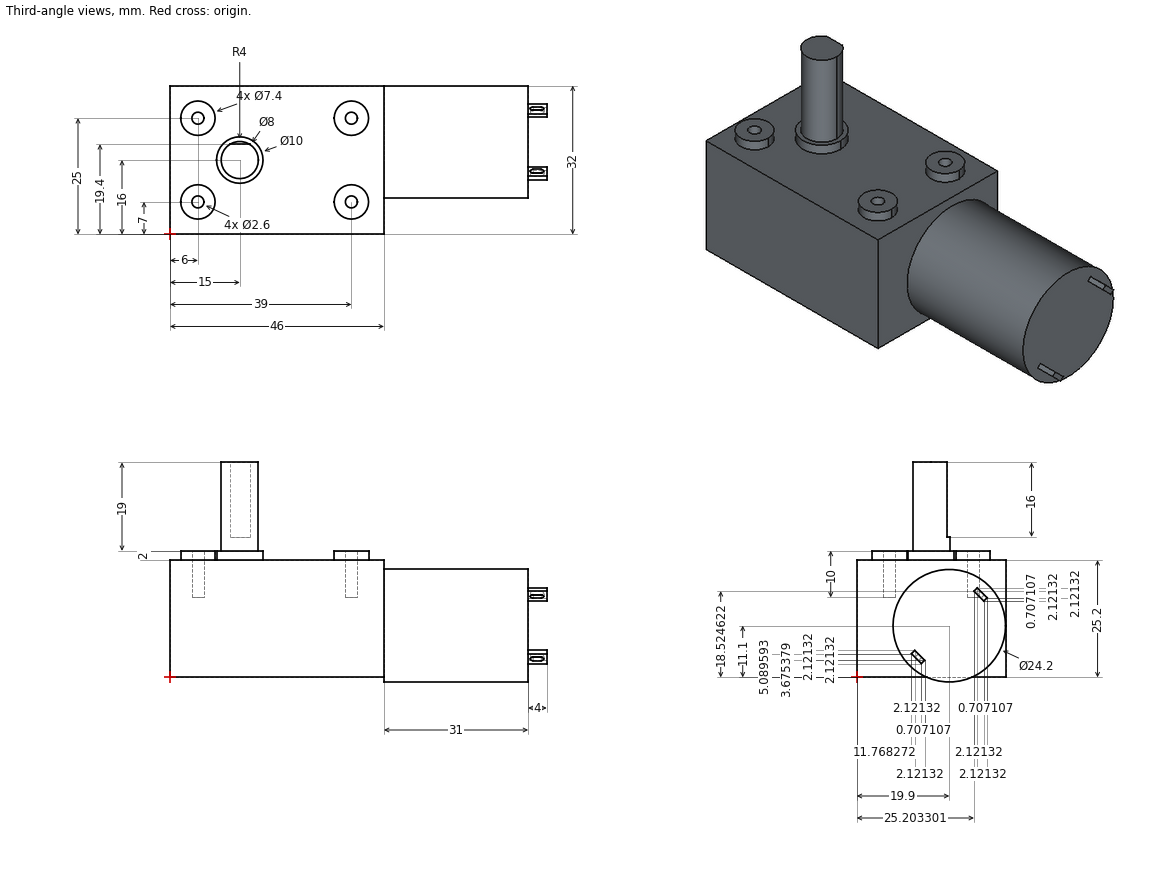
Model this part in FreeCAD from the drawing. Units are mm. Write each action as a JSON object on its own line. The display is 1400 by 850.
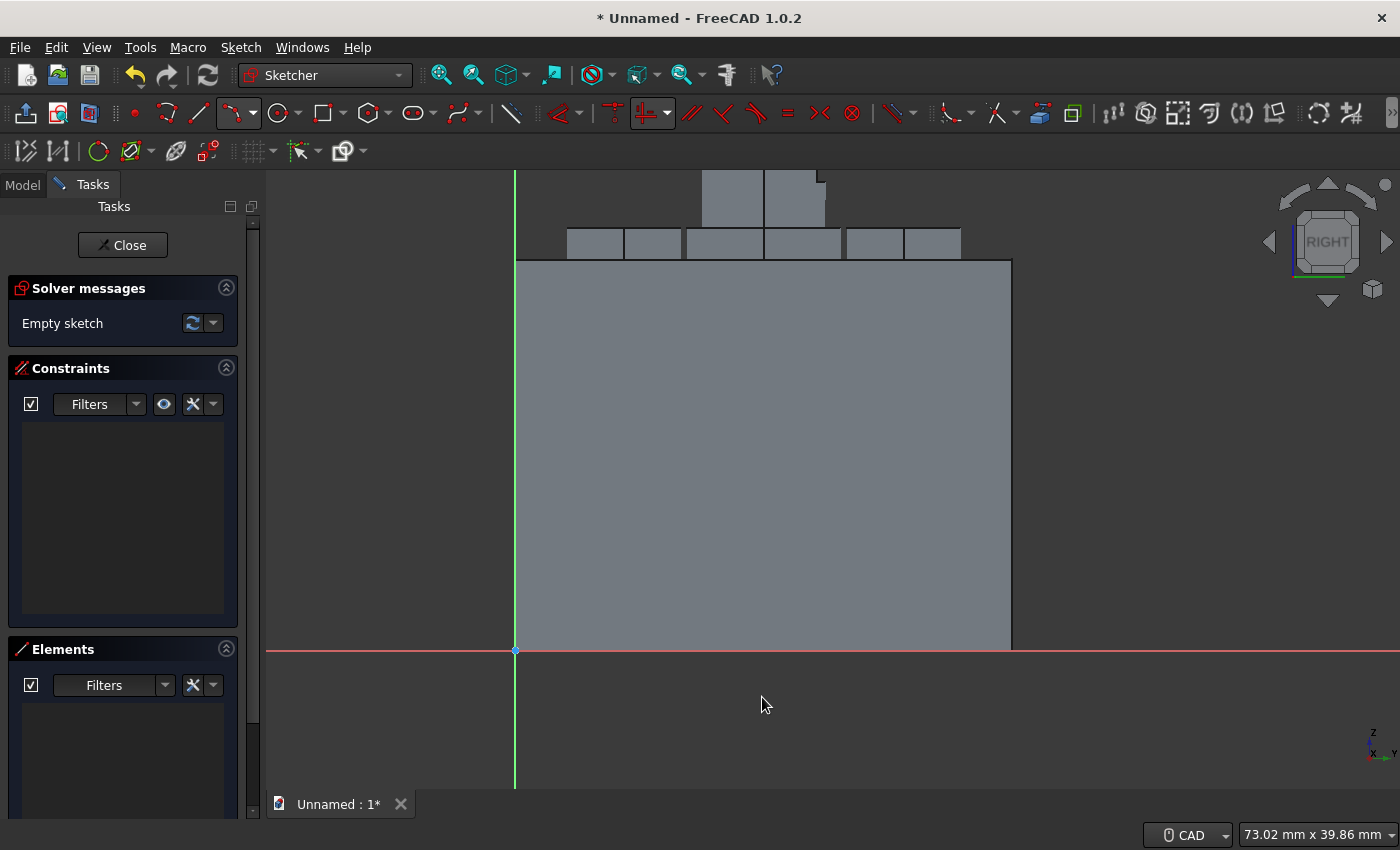
{"action": "left_click", "coordinate": [278, 114]}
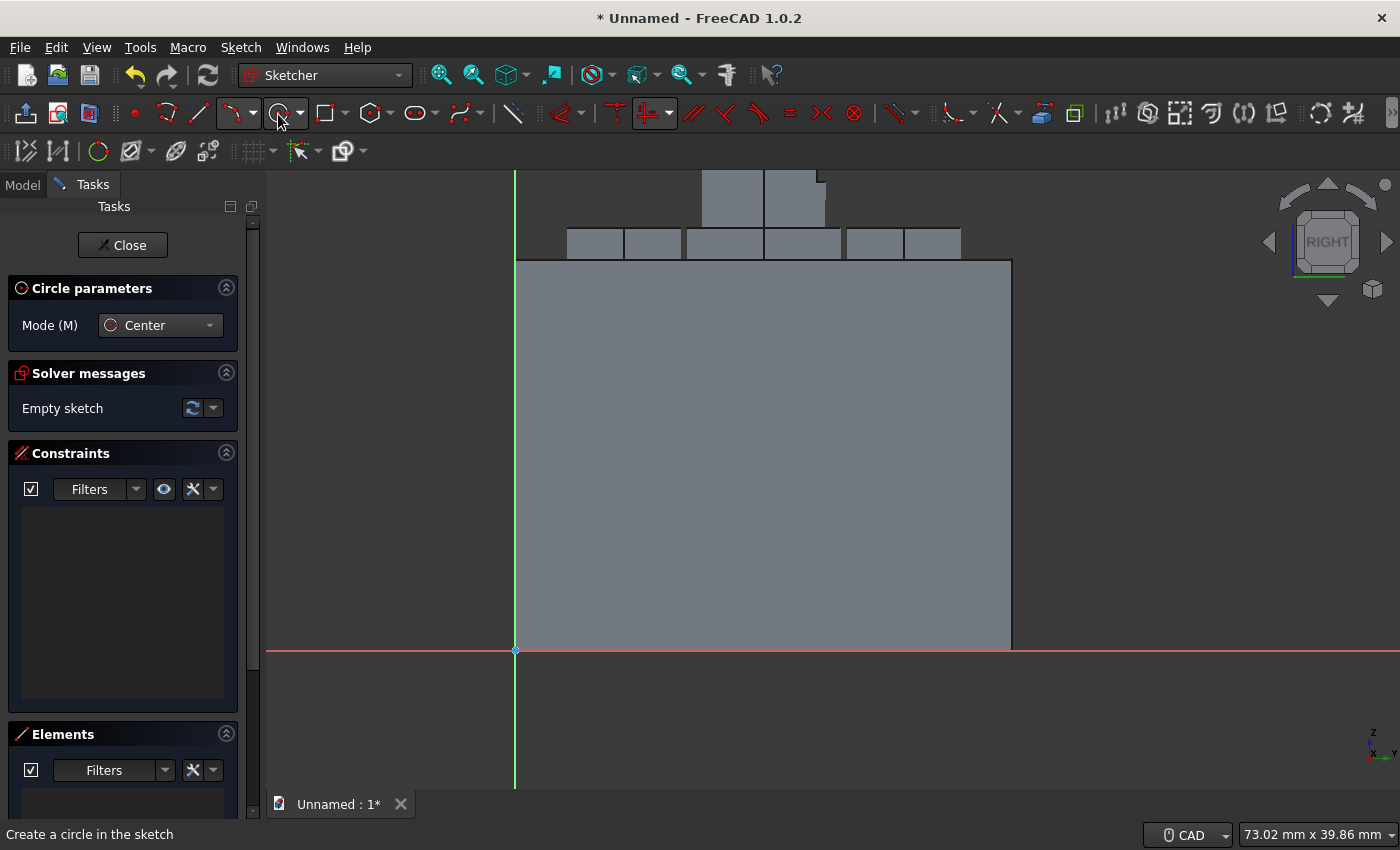
{"action": "left_click", "coordinate": [824, 478]}
{"action": "mouse_move", "coordinate": [957, 346]}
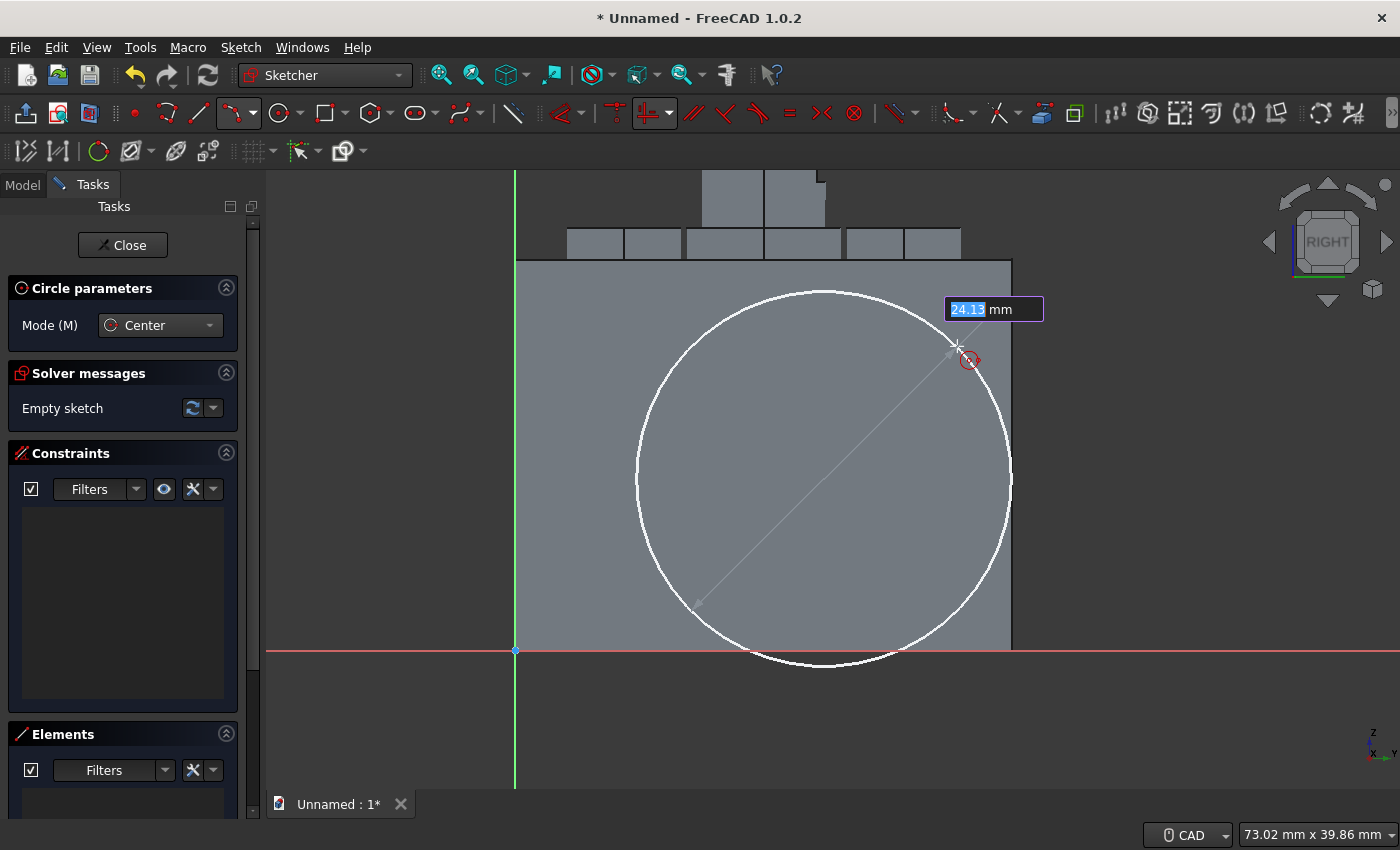
{"action": "type", "text": "24.2"}
{"action": "key", "text": "Return"}
{"action": "key", "text": "Escape"}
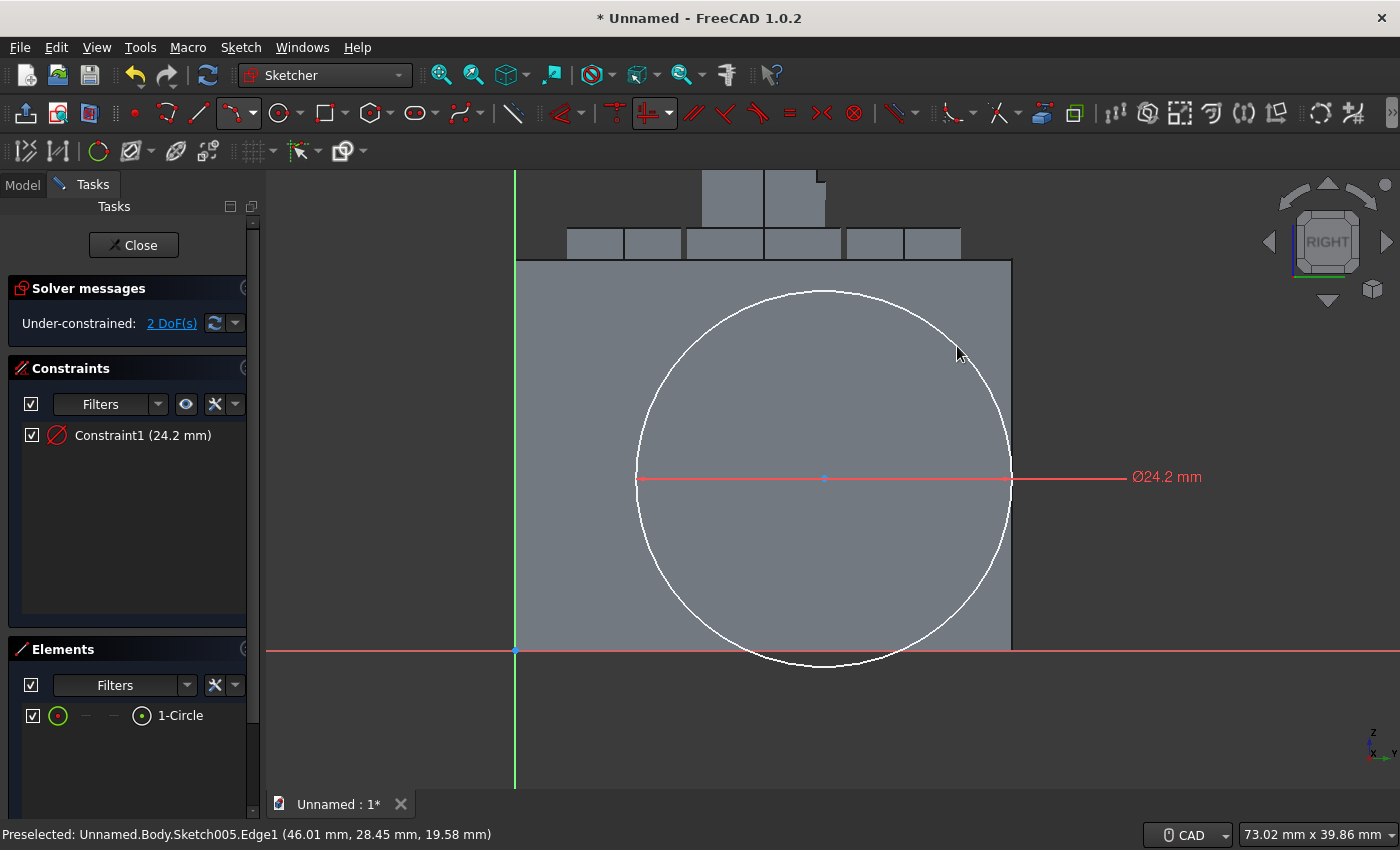
{"action": "left_click", "coordinate": [560, 114]}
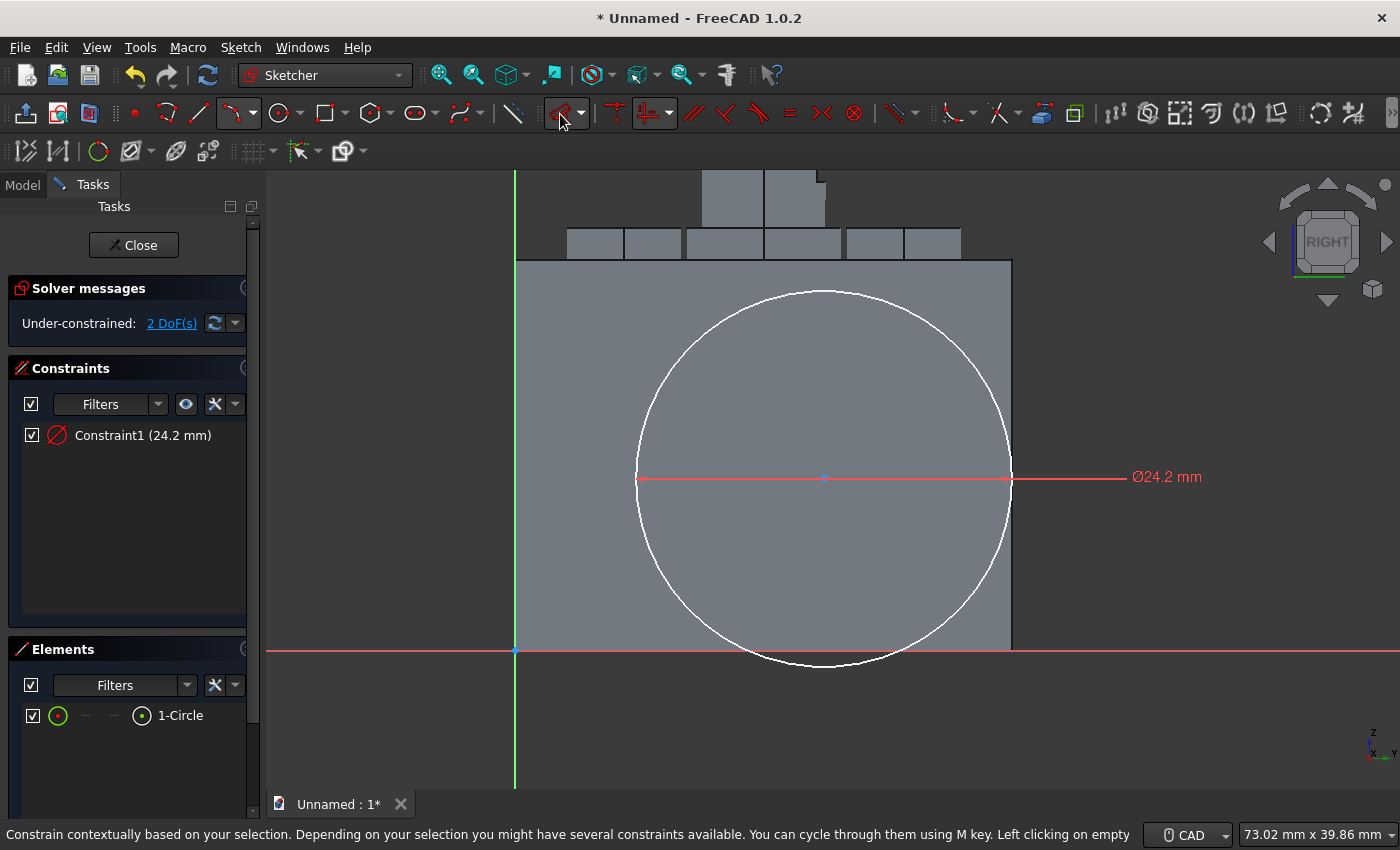
{"action": "left_click", "coordinate": [824, 479]}
{"action": "left_click", "coordinate": [670, 685]}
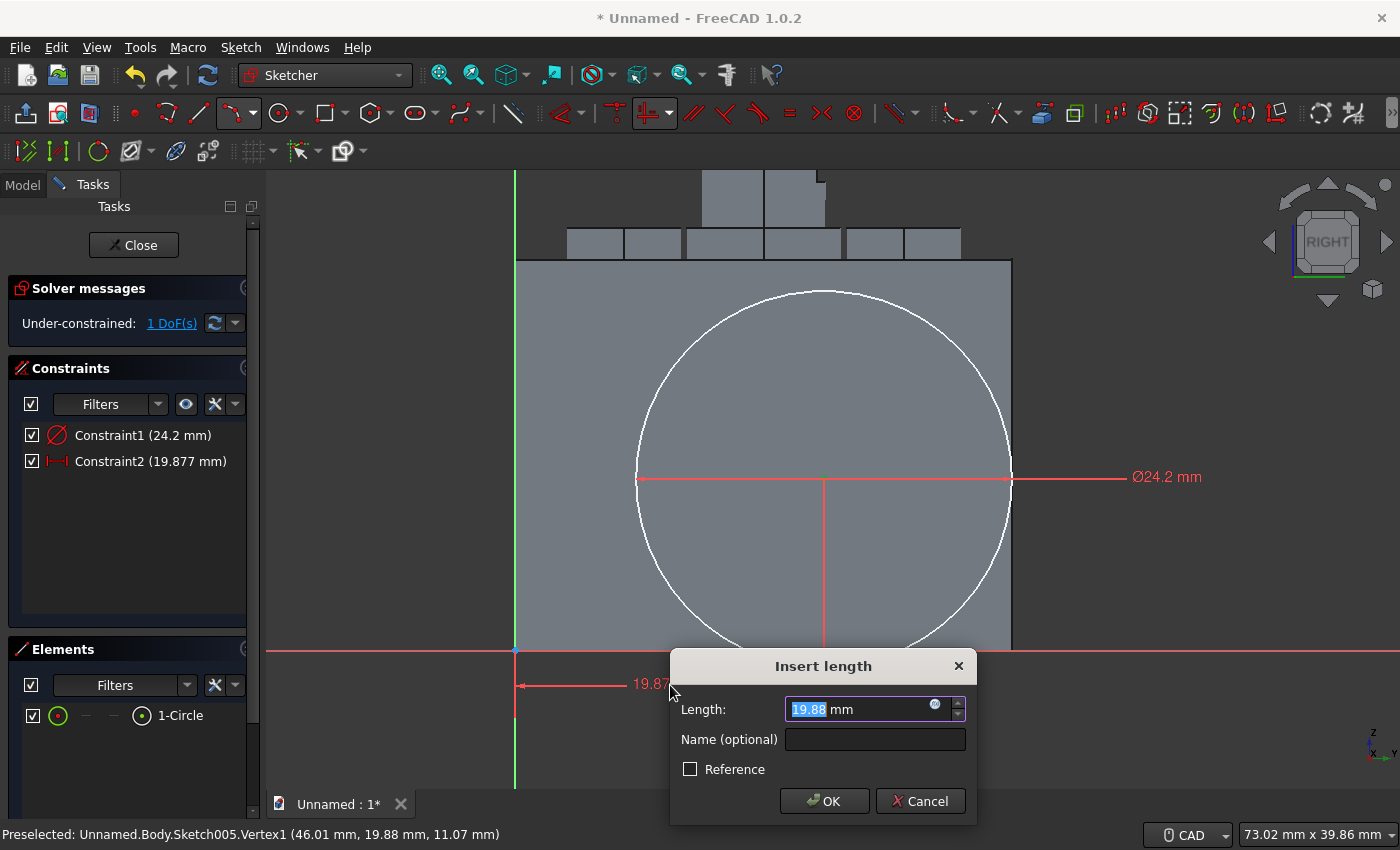
{"action": "type", "text": "19.9"}
{"action": "key", "text": "Return"}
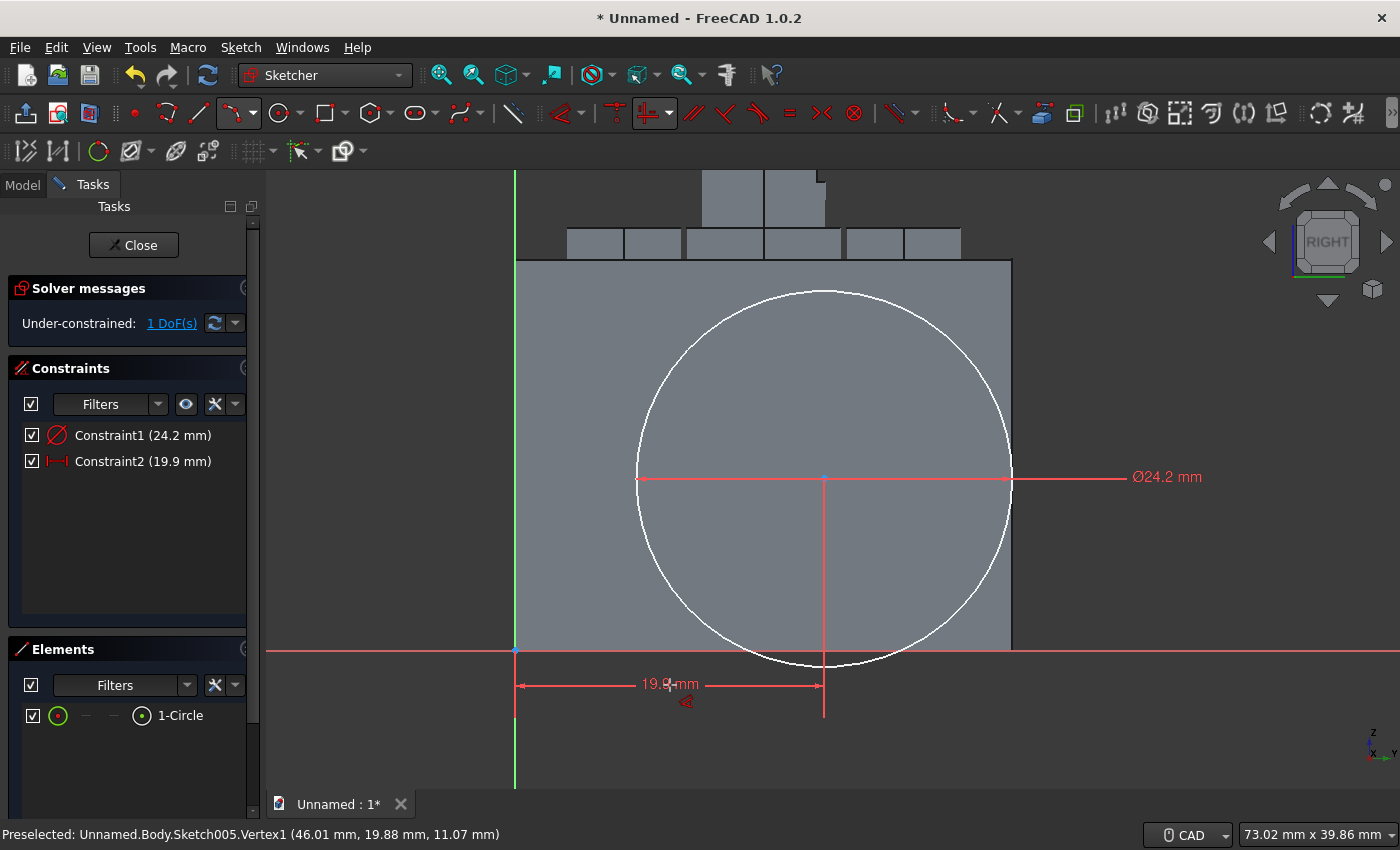
{"action": "left_click", "coordinate": [824, 479]}
{"action": "left_click", "coordinate": [481, 565]}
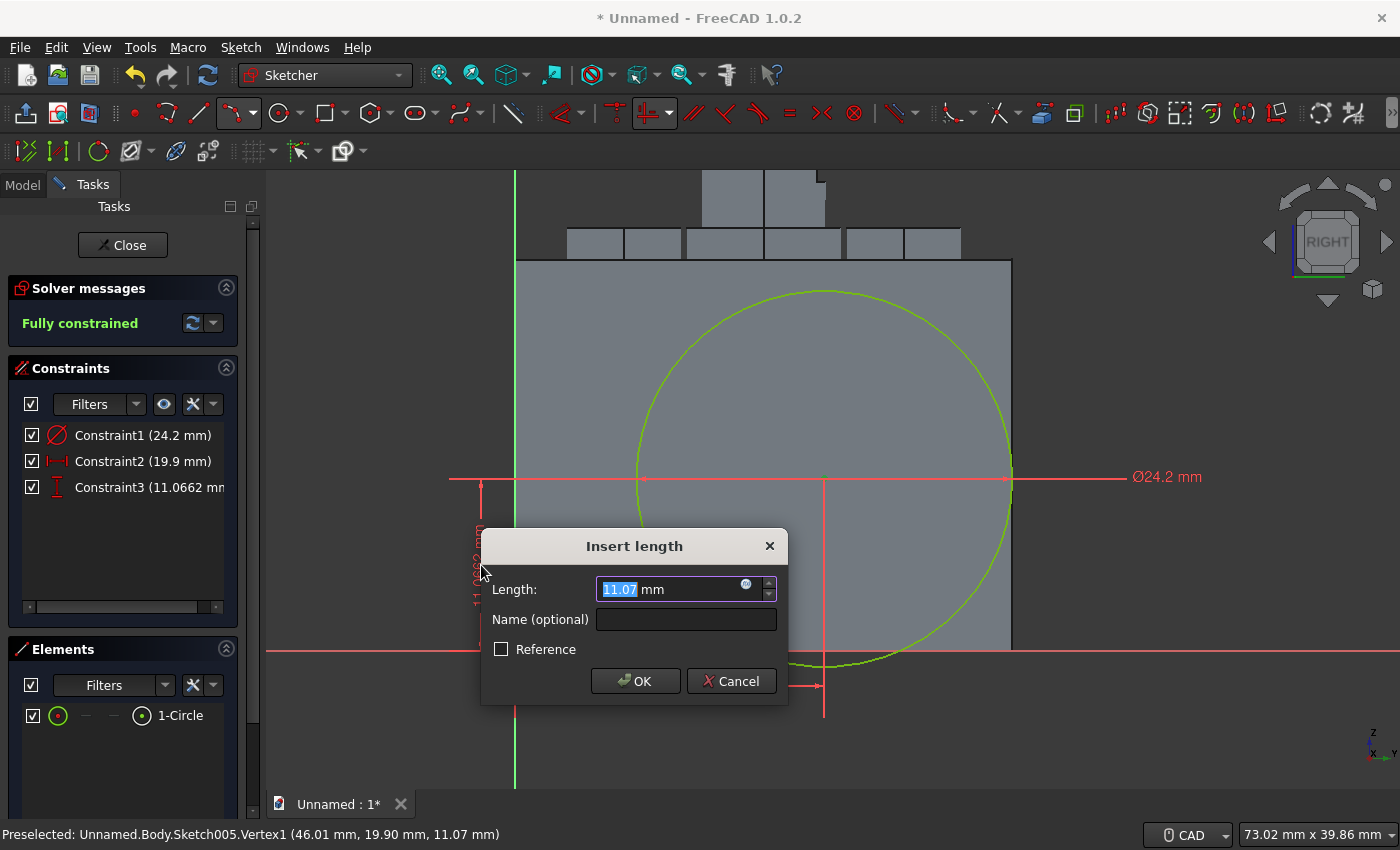
{"action": "type", "text": "11.1"}
{"action": "key", "text": "Return"}
{"action": "key", "text": "Escape"}